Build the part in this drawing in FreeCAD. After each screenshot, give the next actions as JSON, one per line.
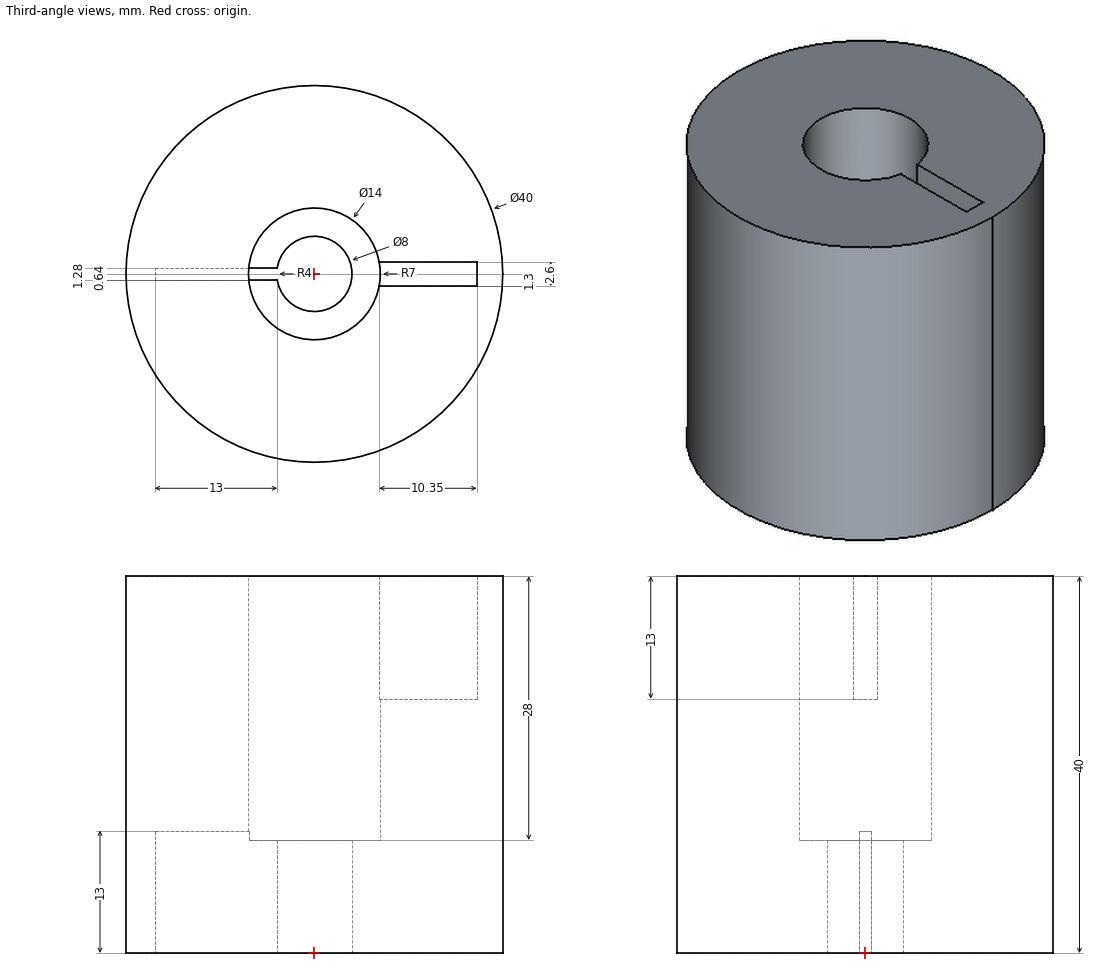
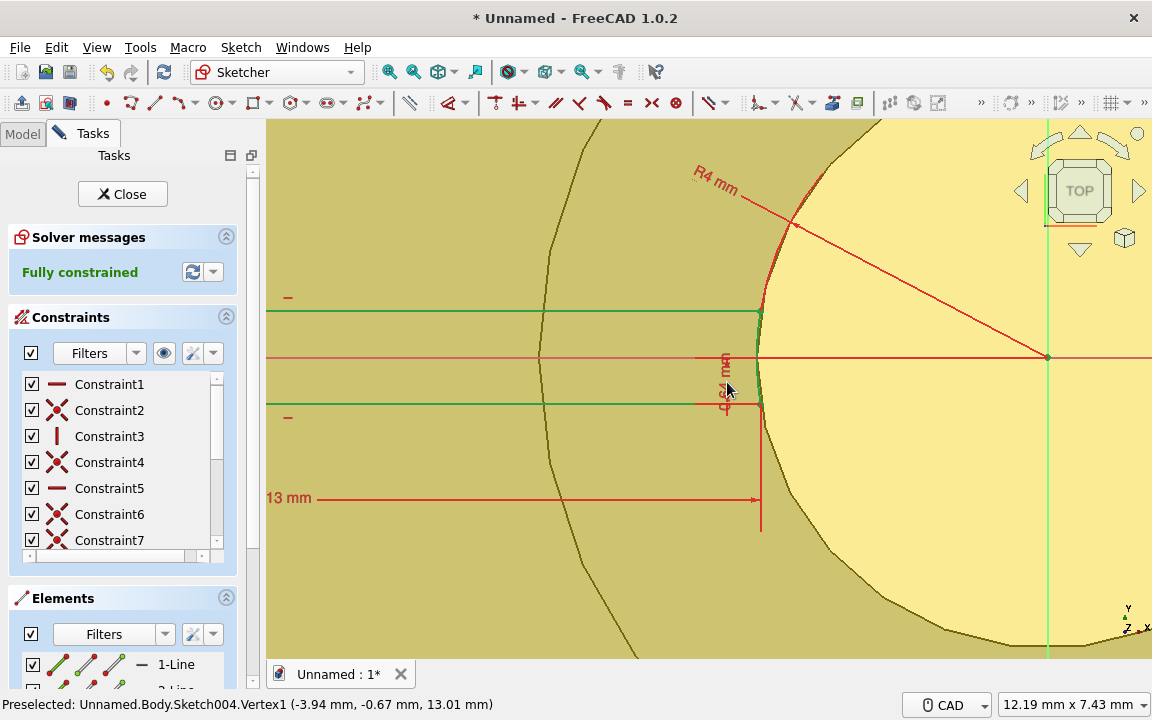
{"action": "left_click", "coordinate": [123, 194]}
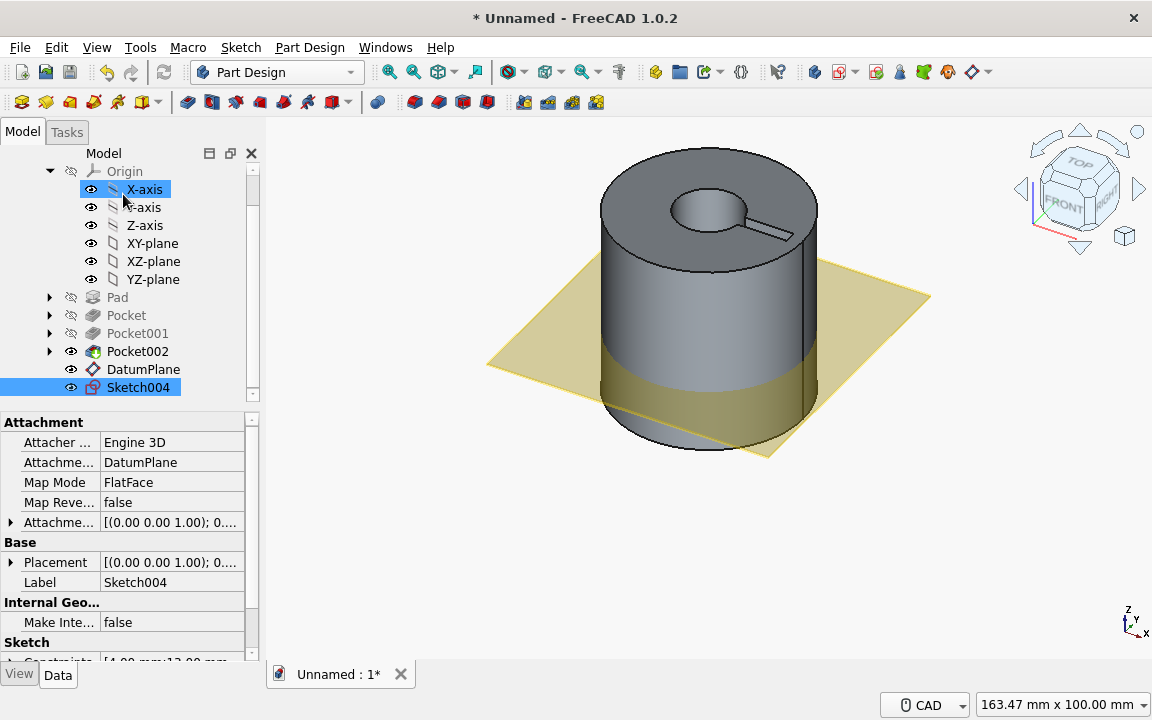
{"action": "left_click", "coordinate": [188, 102]}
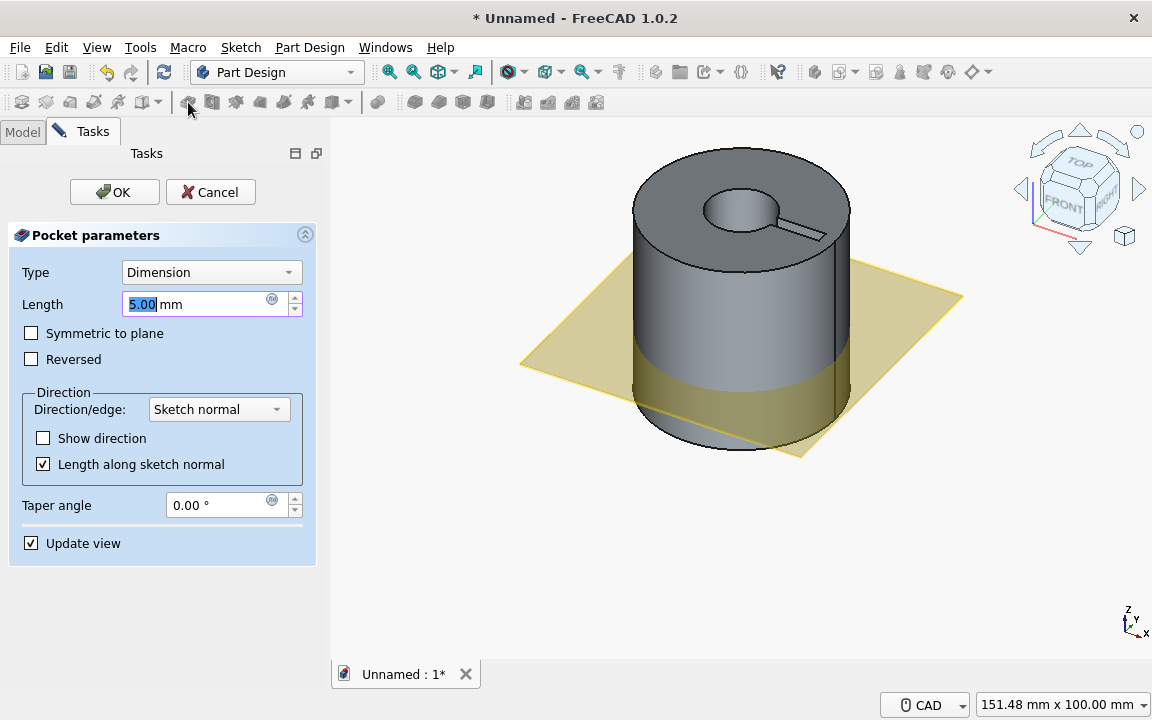
{"action": "type", "text": "13"}
{"action": "key", "text": "Tab"}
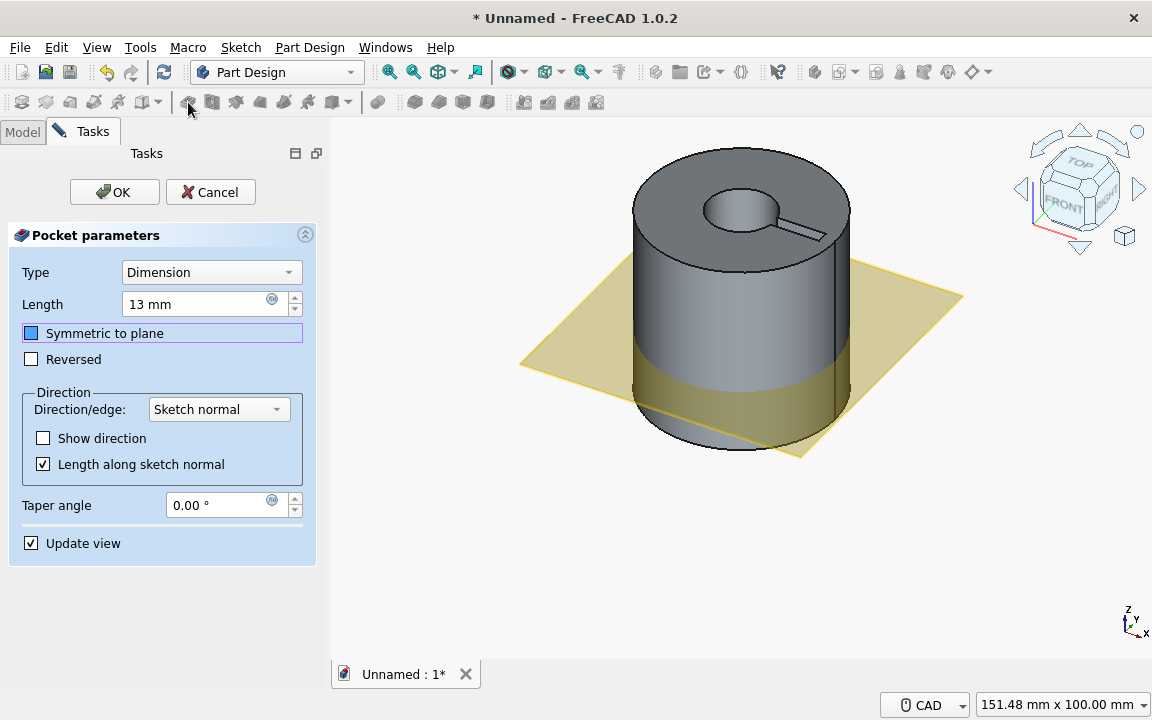
{"action": "left_click", "coordinate": [115, 192]}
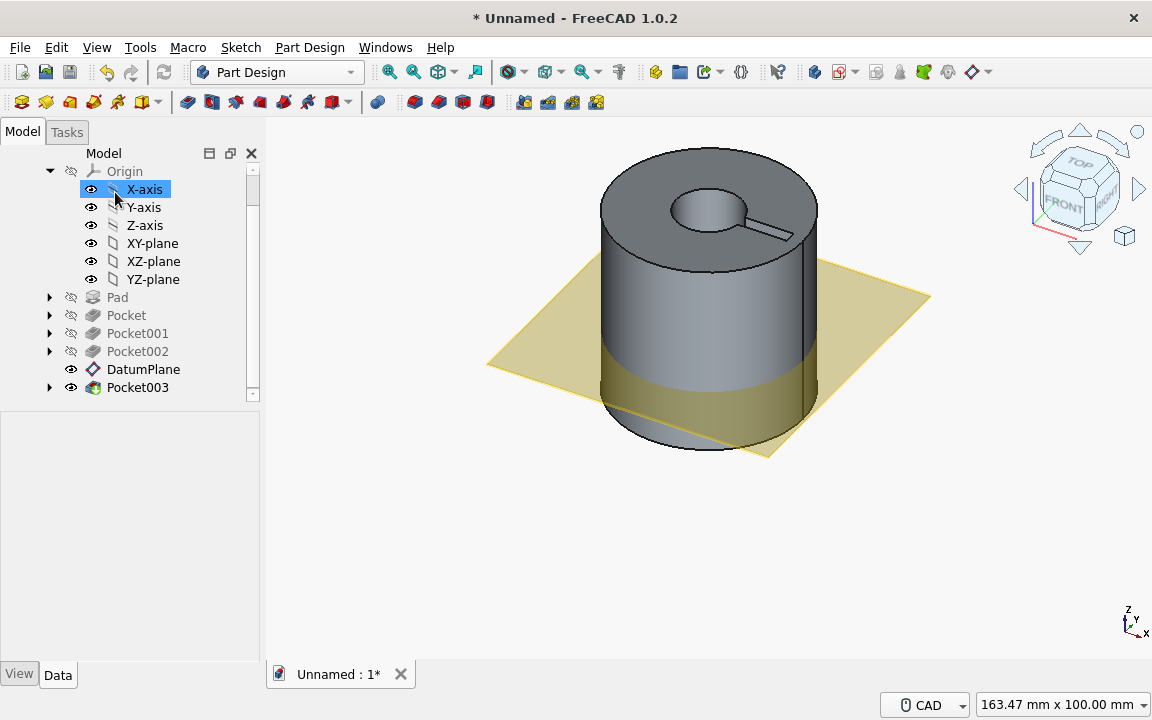
{"action": "left_click", "coordinate": [116, 369]}
{"action": "key", "text": "space"}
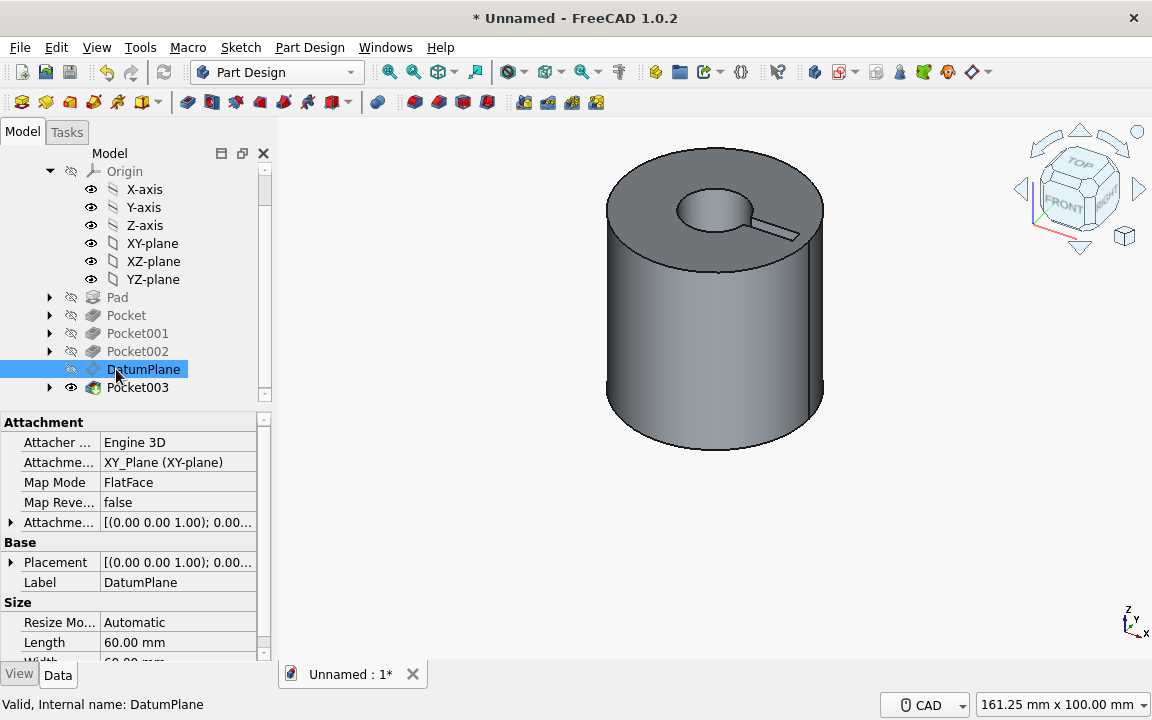
{"action": "key", "text": "0"}